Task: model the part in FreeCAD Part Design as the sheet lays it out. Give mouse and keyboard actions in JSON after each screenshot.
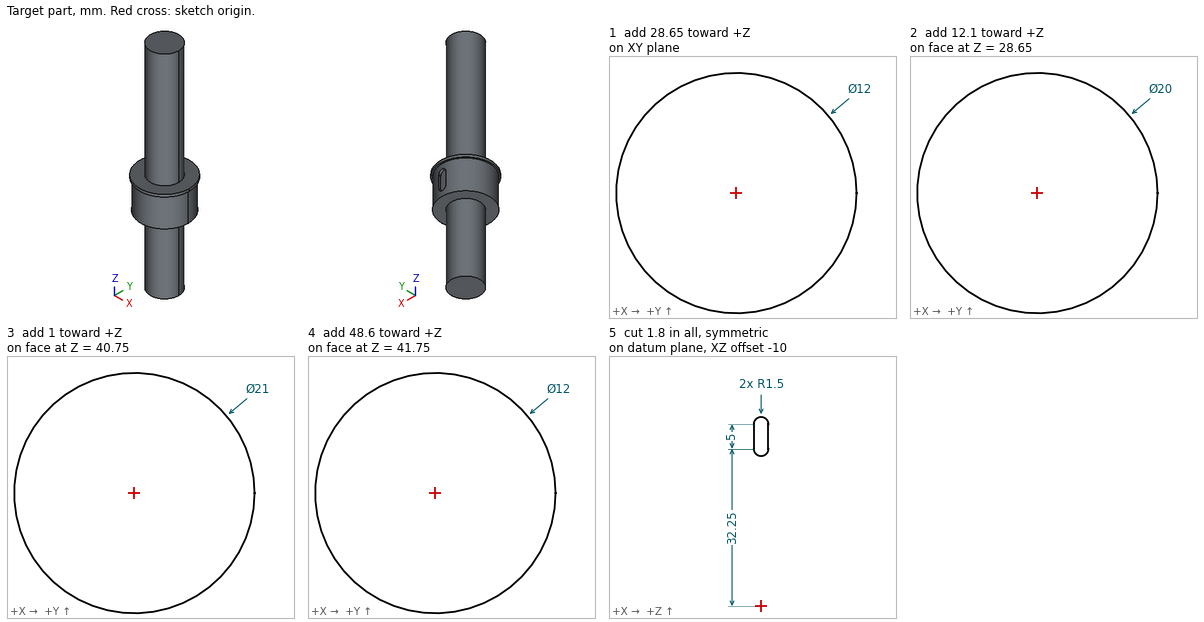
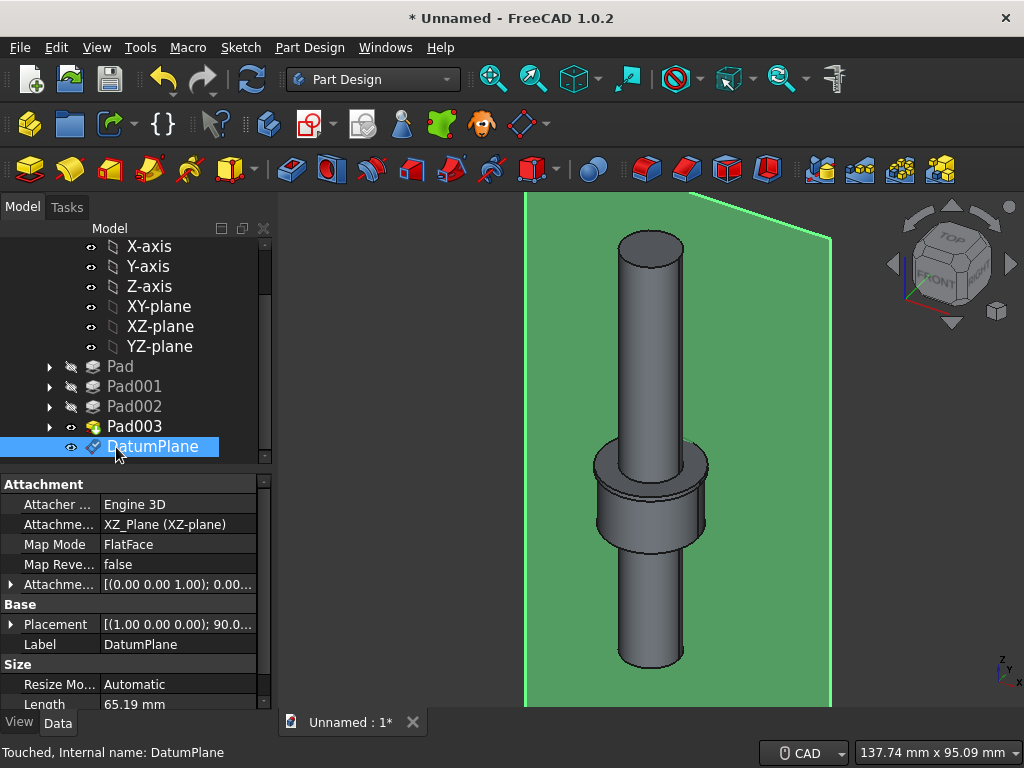
{"action": "left_click", "coordinate": [310, 124]}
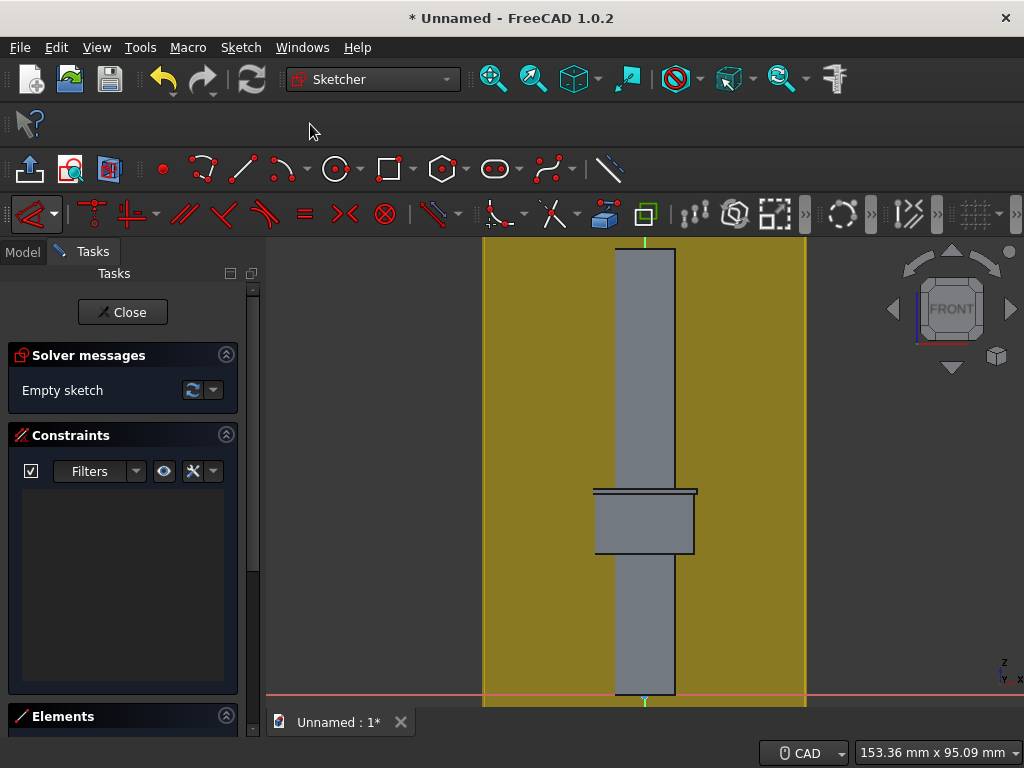
{"action": "left_click", "coordinate": [110, 170]}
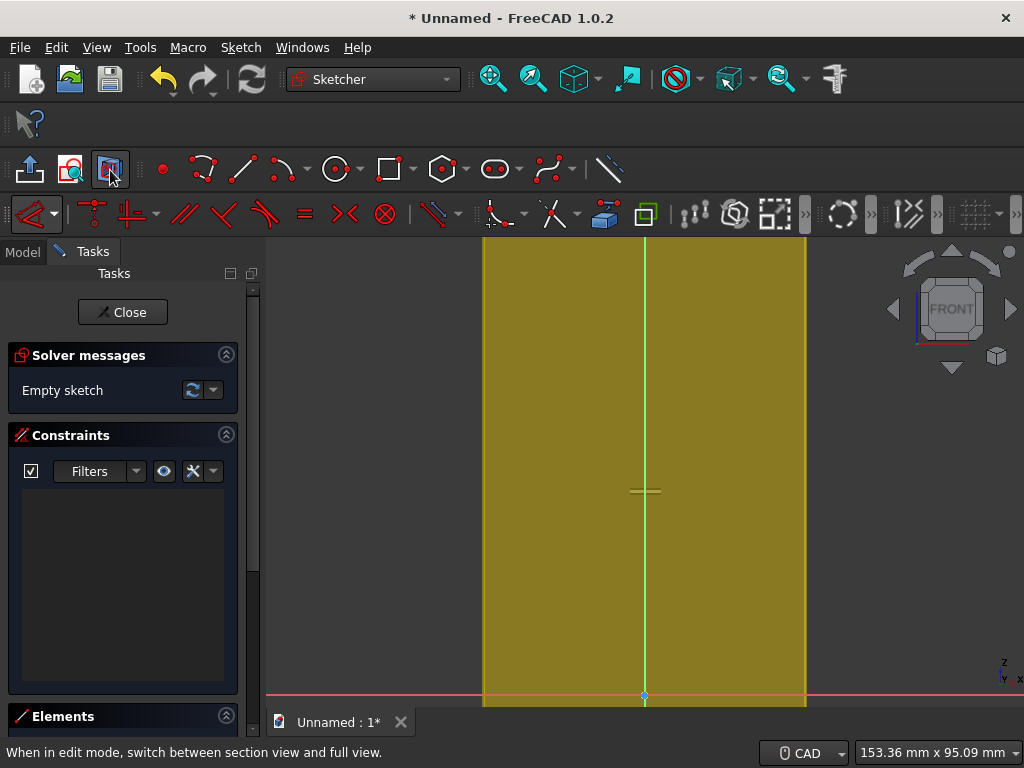
{"action": "scroll", "coordinate": [656, 532], "scroll_direction": "up", "scroll_amount": 10}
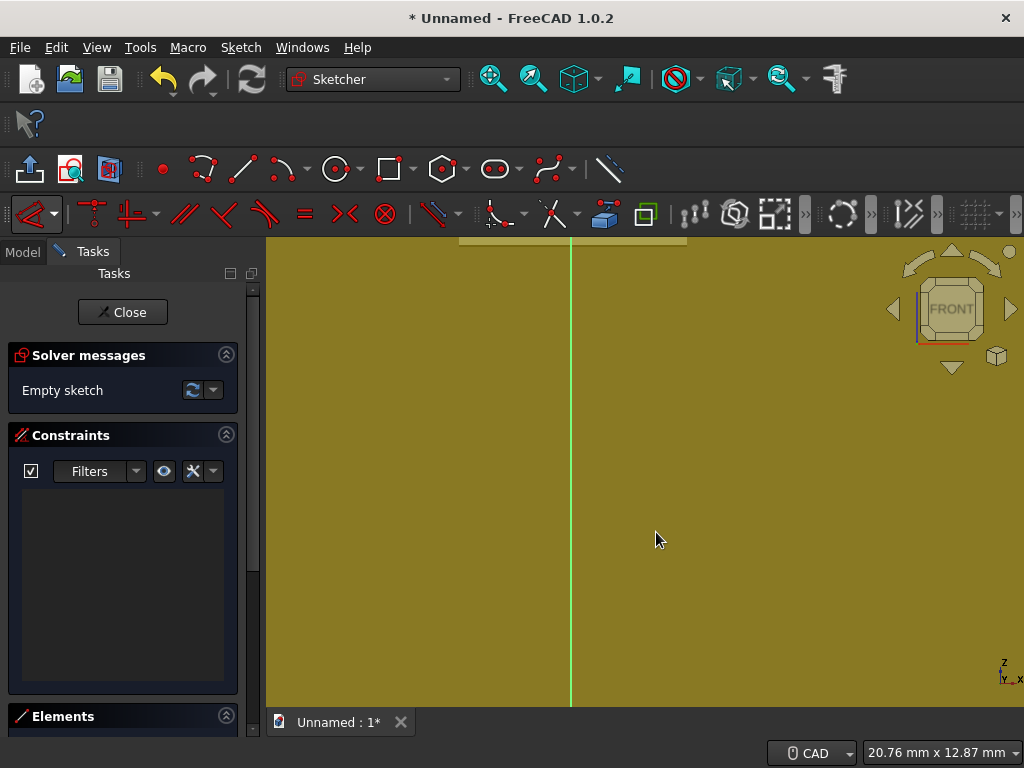
{"action": "left_click", "coordinate": [496, 170]}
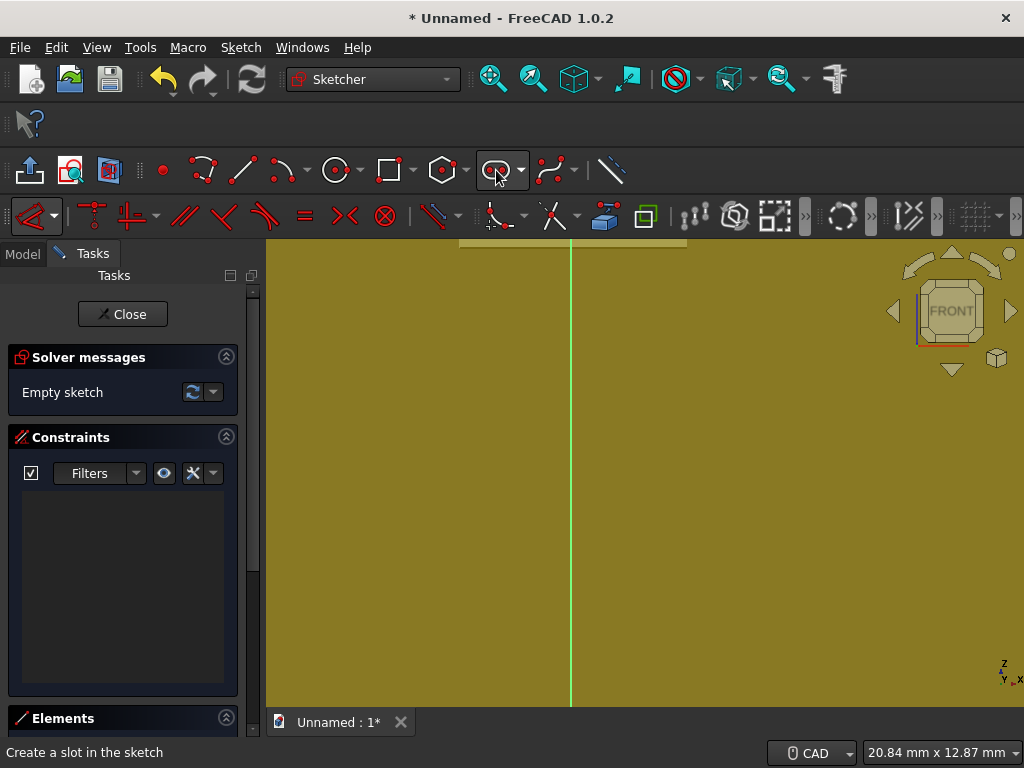
{"action": "left_click", "coordinate": [571, 557]}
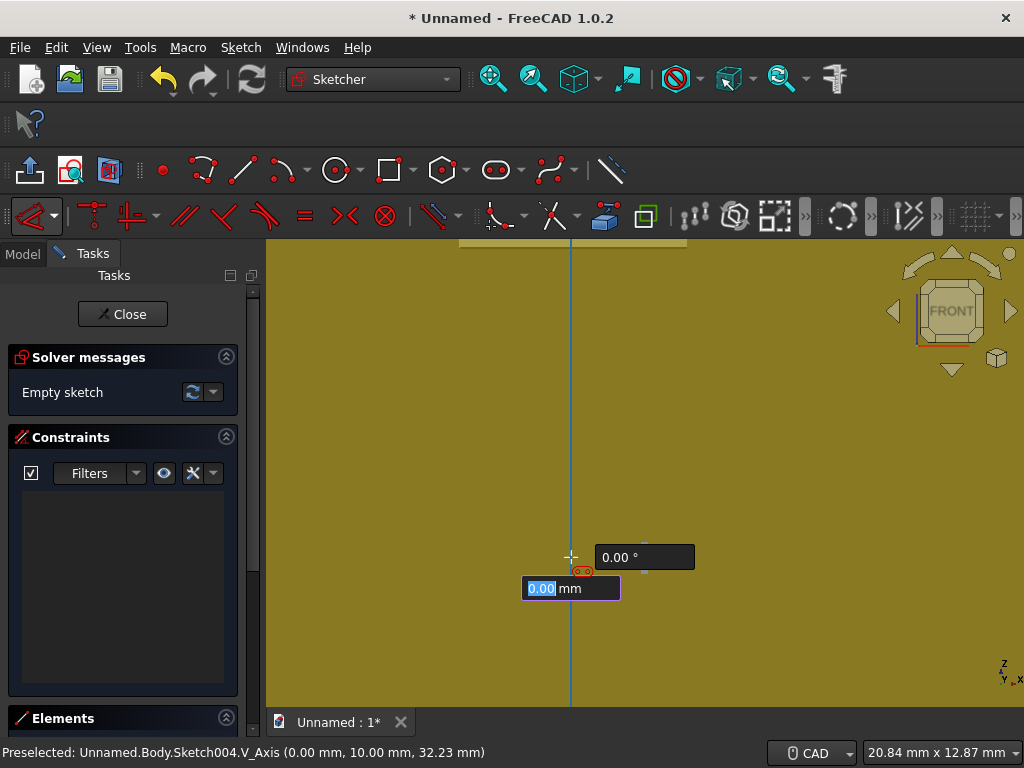
{"action": "left_click", "coordinate": [580, 375]}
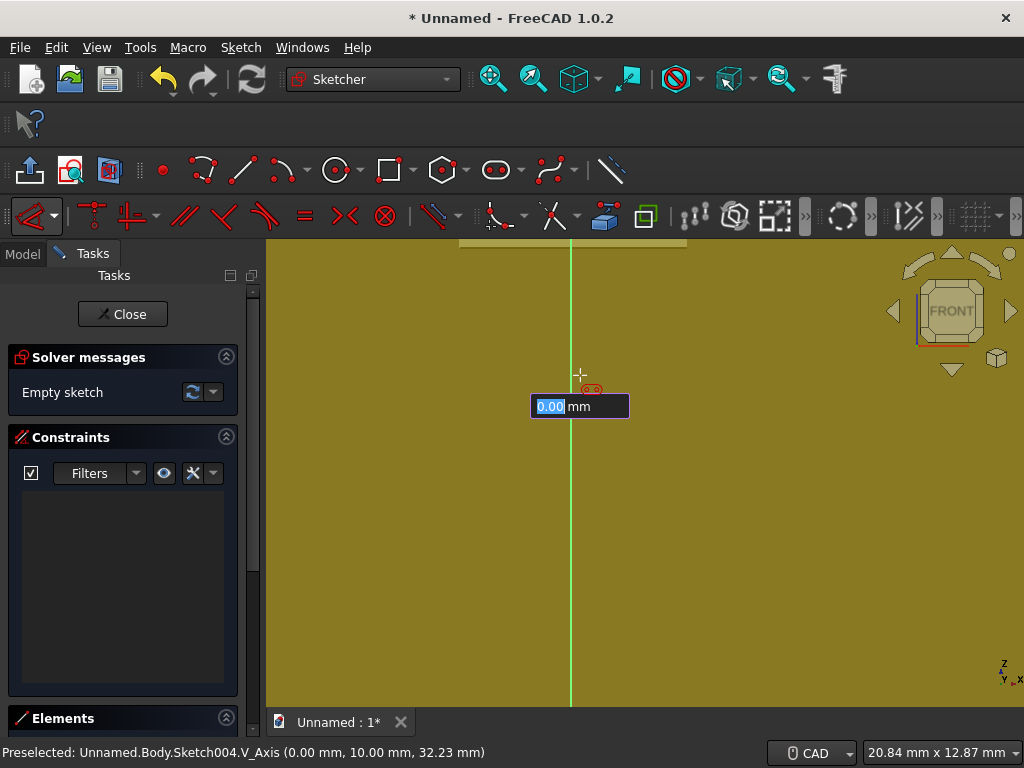
{"action": "left_click", "coordinate": [626, 466]}
{"action": "key", "text": "Escape"}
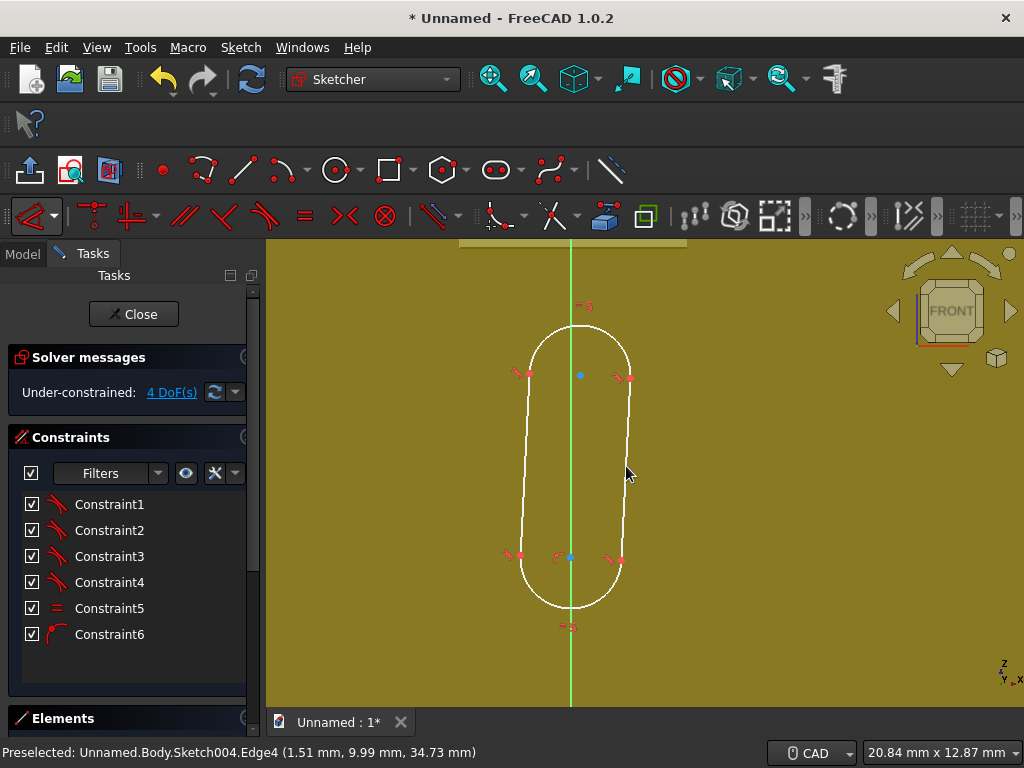
{"action": "left_click", "coordinate": [523, 501]}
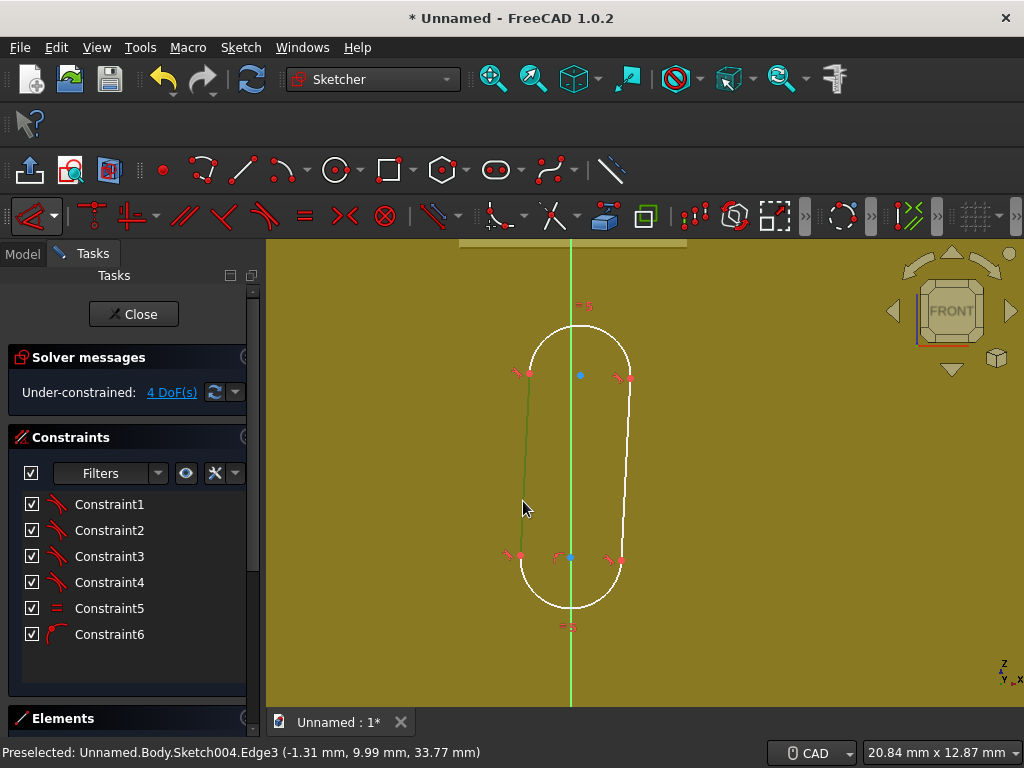
{"action": "left_click", "coordinate": [158, 216]}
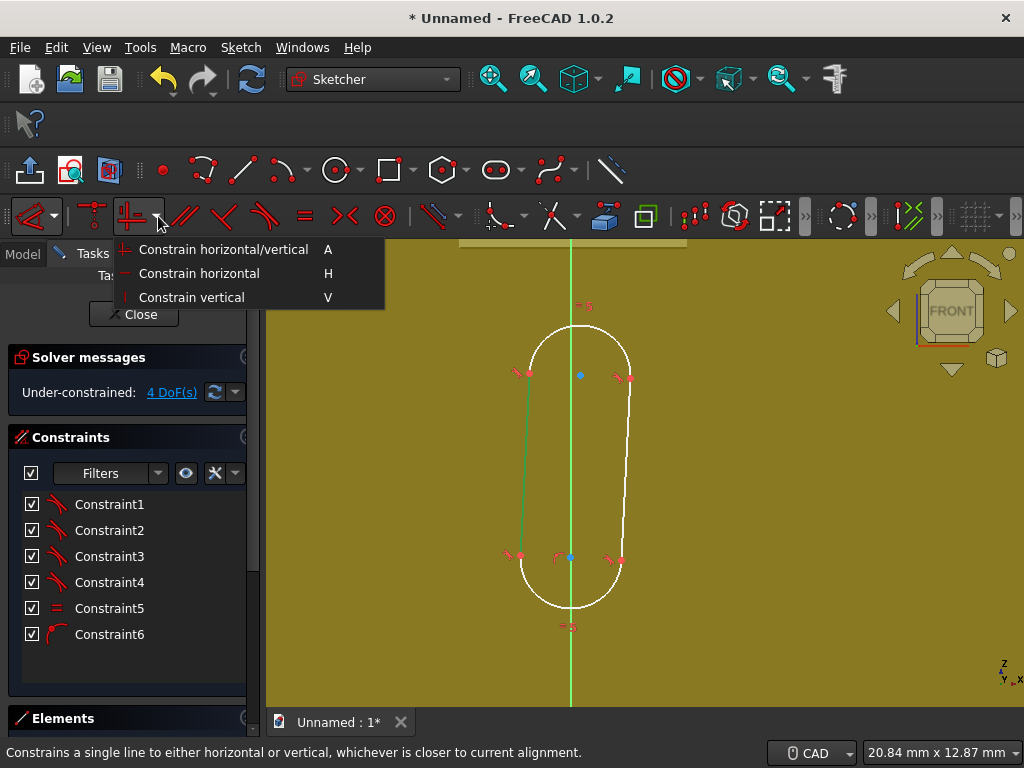
{"action": "left_click", "coordinate": [249, 297]}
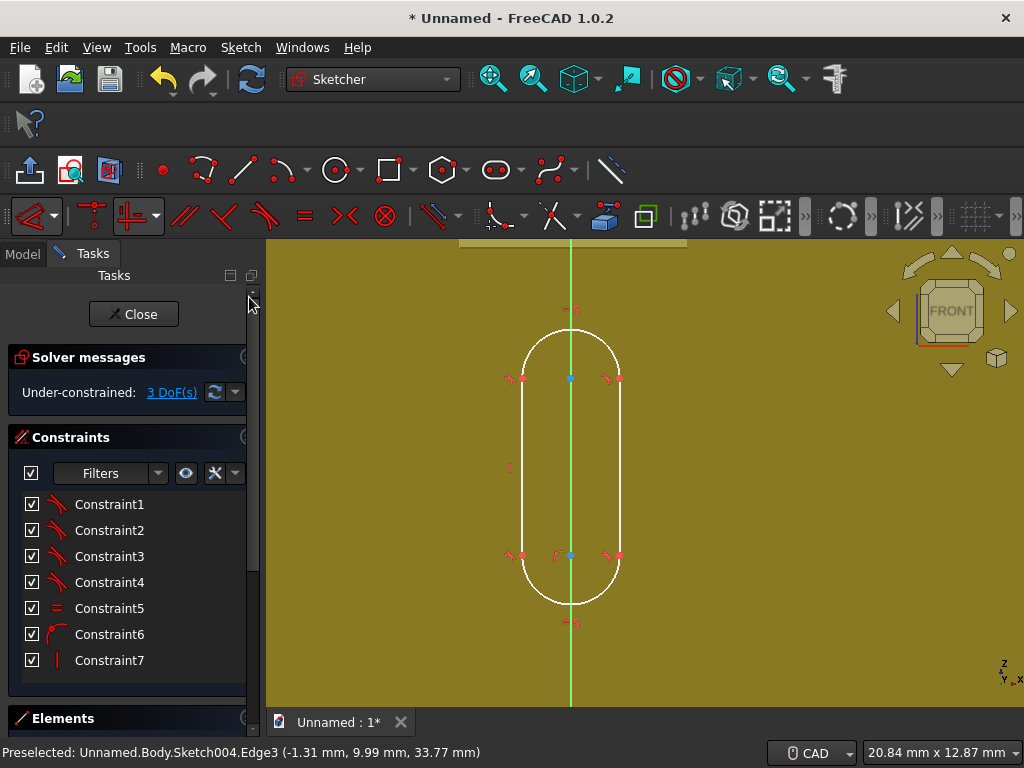
{"action": "left_click", "coordinate": [542, 595]}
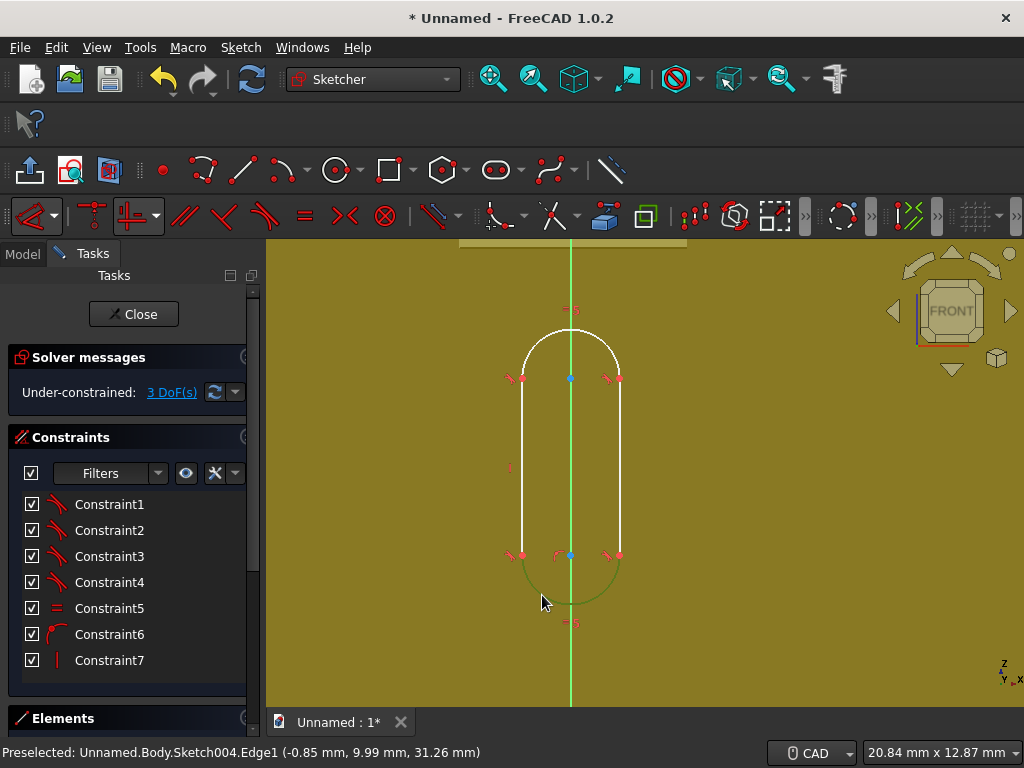
{"action": "left_click", "coordinate": [56, 216]}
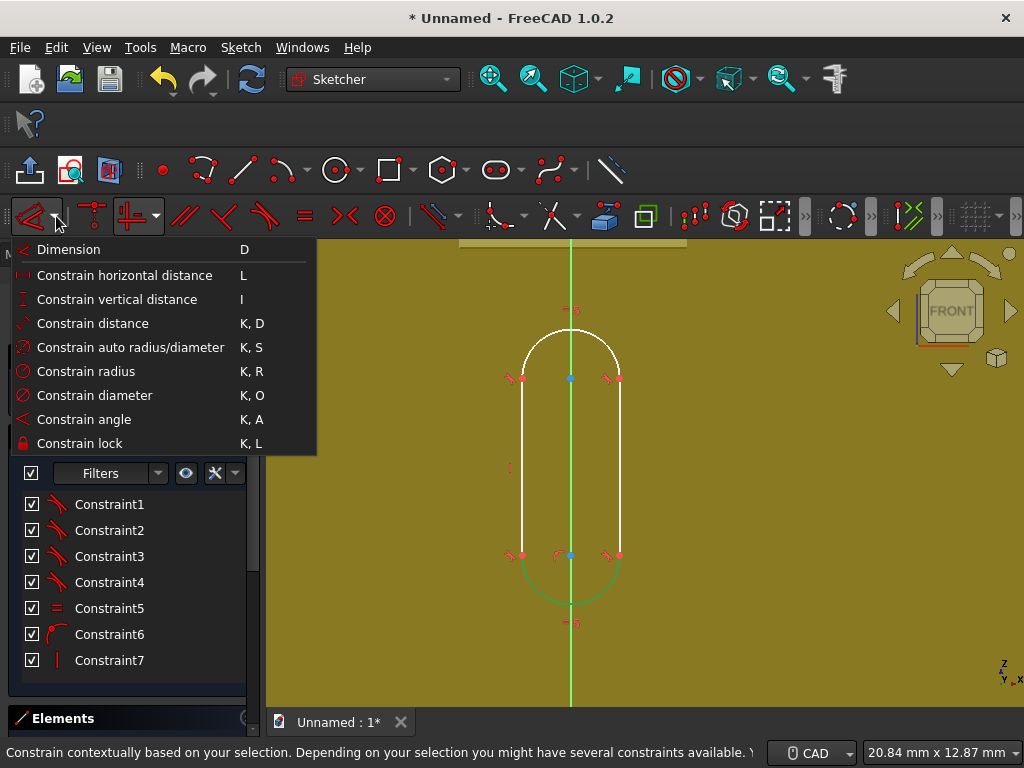
{"action": "left_click", "coordinate": [164, 371]}